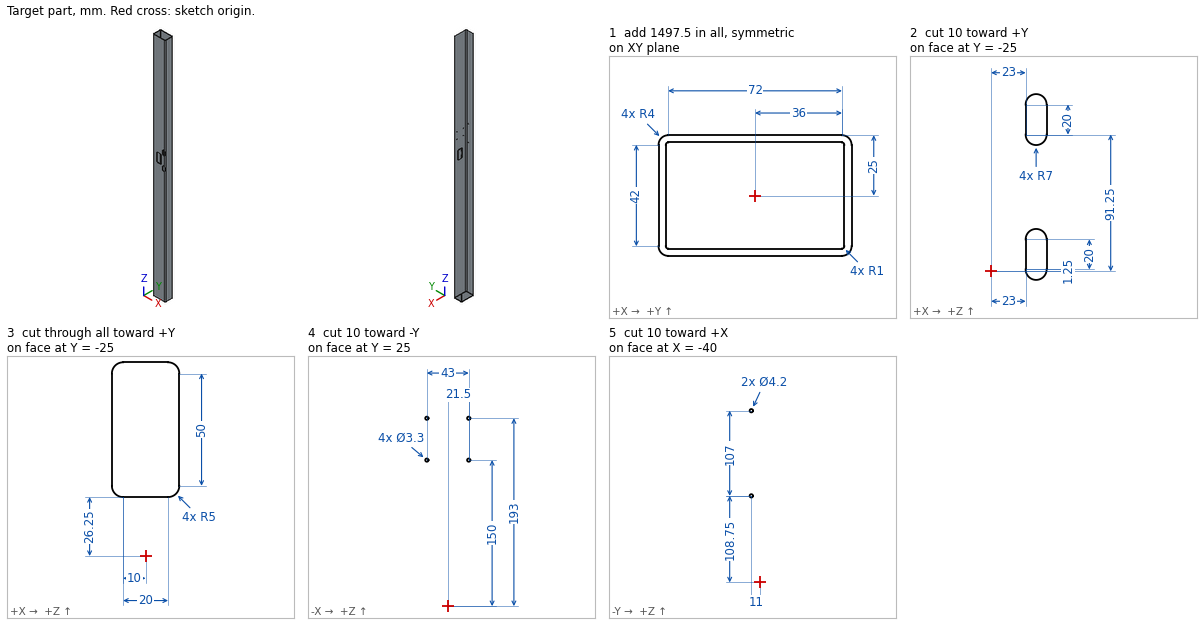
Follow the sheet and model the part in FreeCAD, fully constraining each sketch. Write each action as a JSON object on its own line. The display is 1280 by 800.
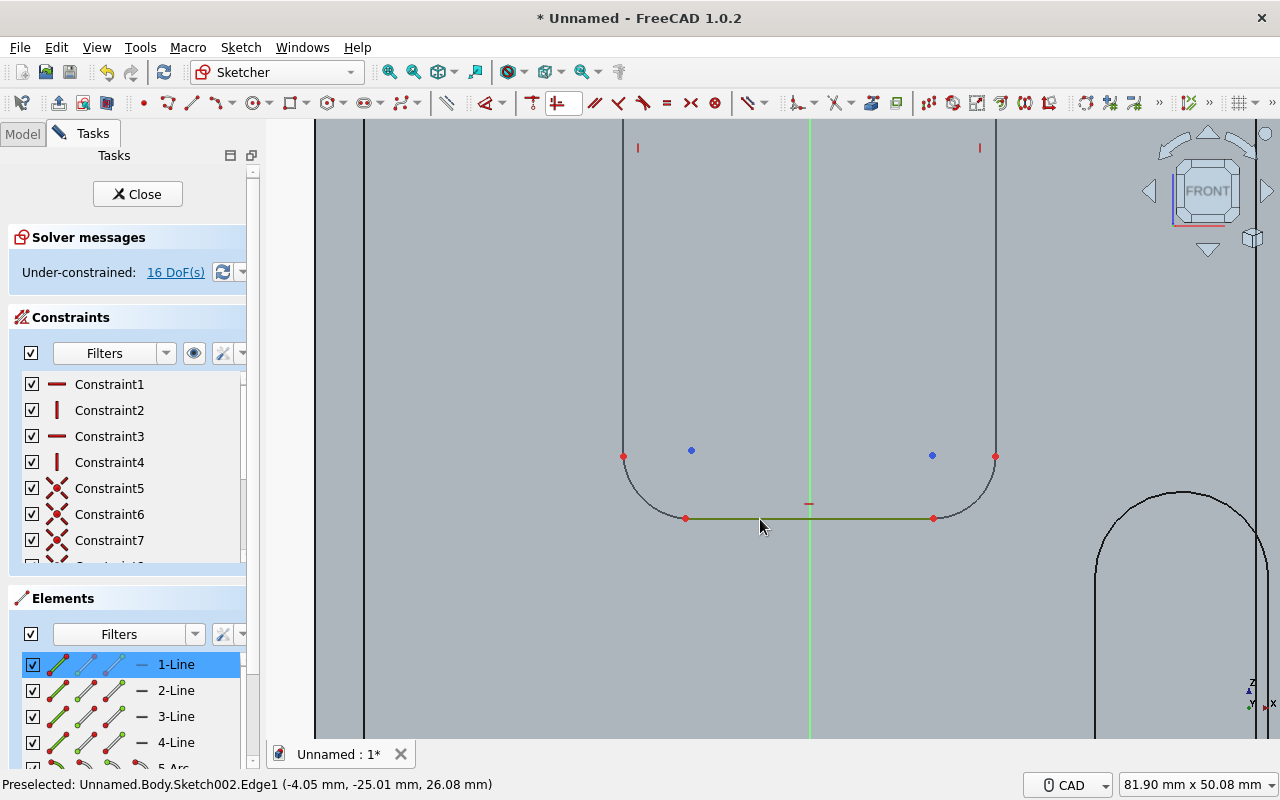
{"action": "left_click", "coordinate": [961, 512]}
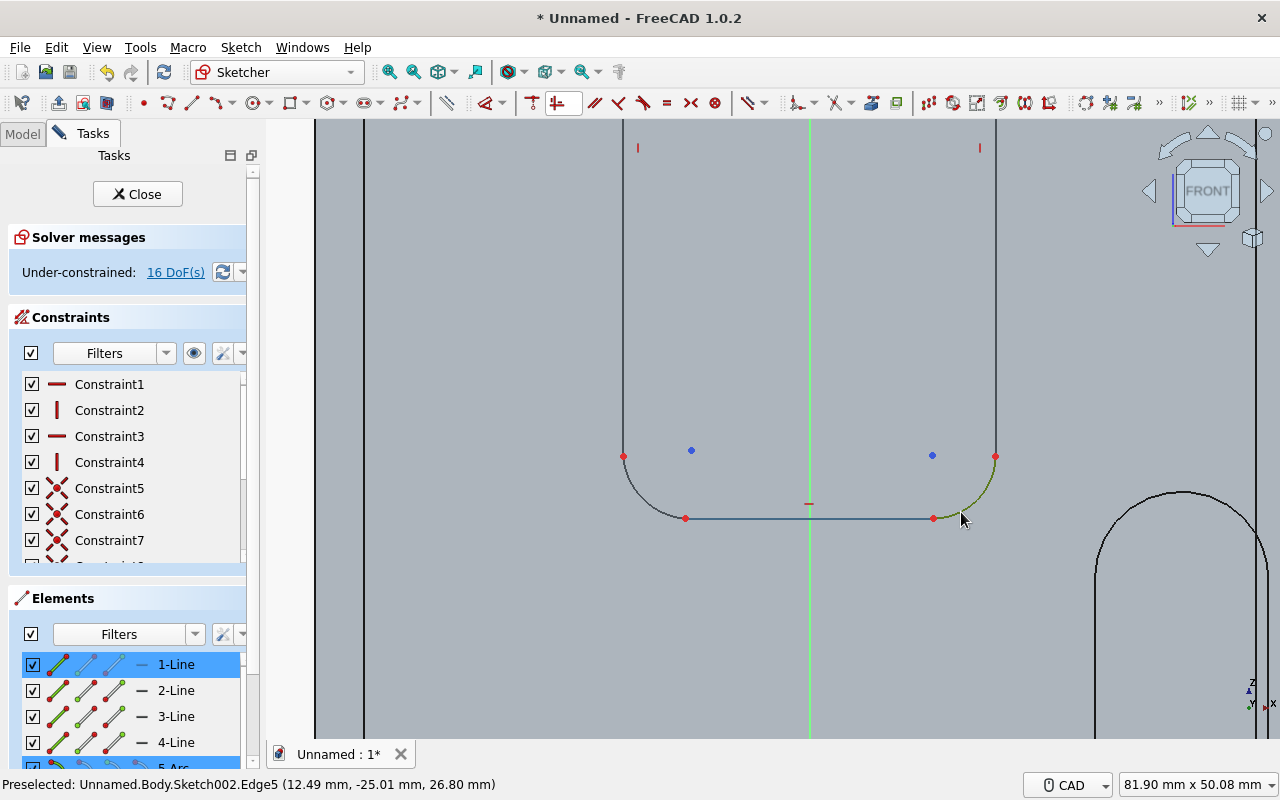
{"action": "key", "text": "t"}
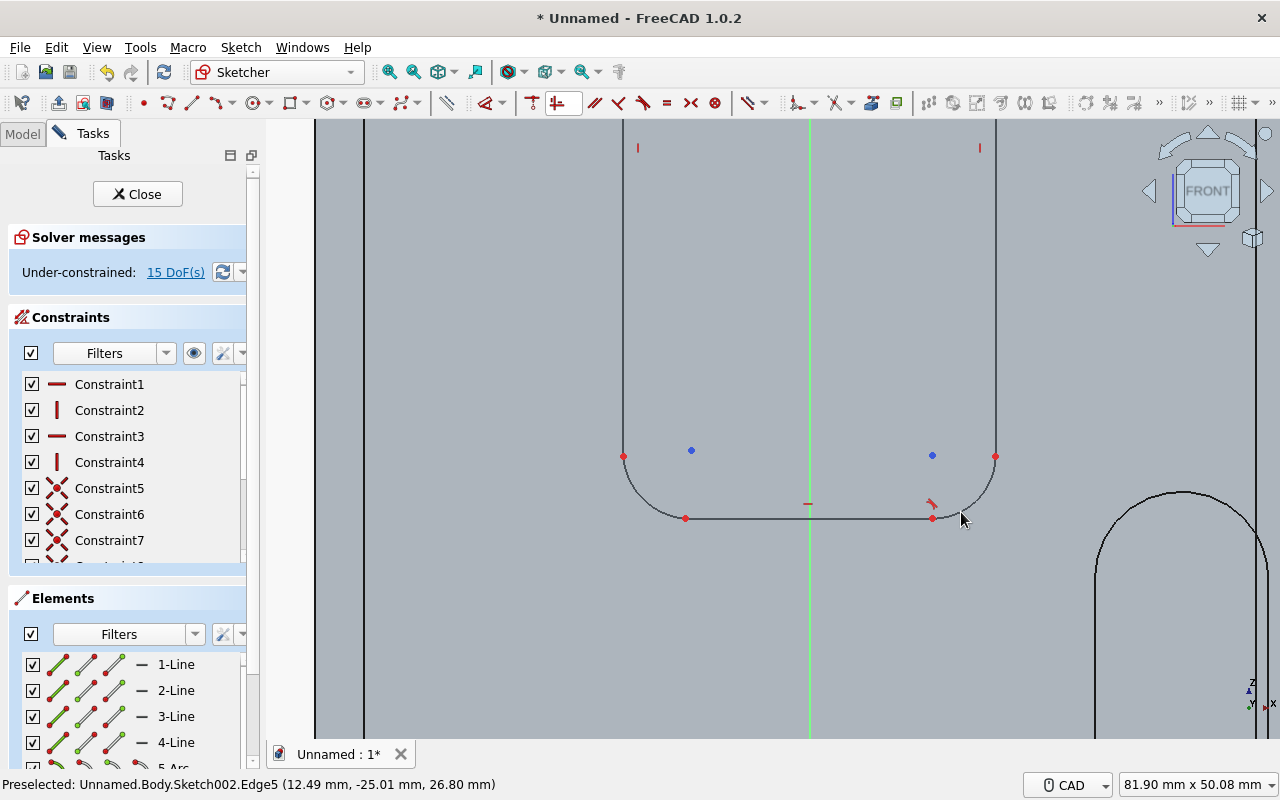
{"action": "left_click", "coordinate": [760, 519]}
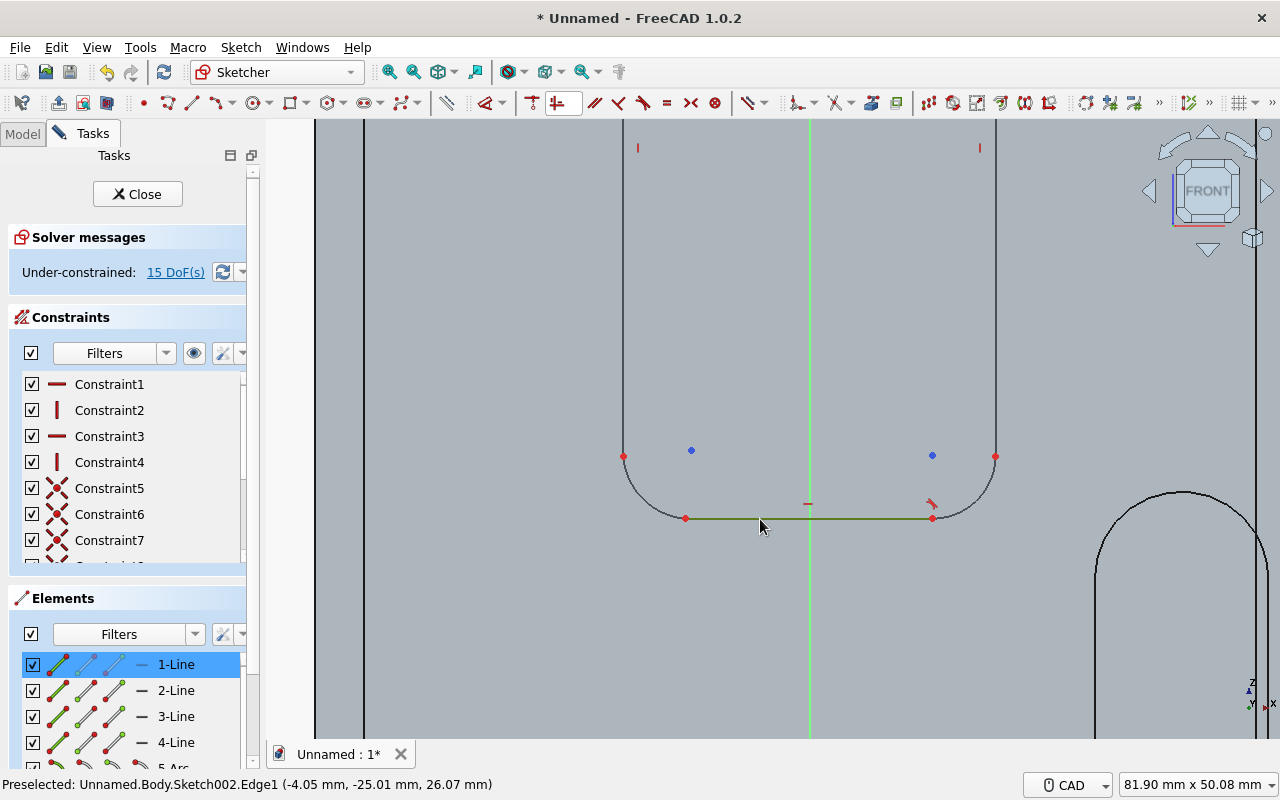
{"action": "left_click", "coordinate": [631, 484]}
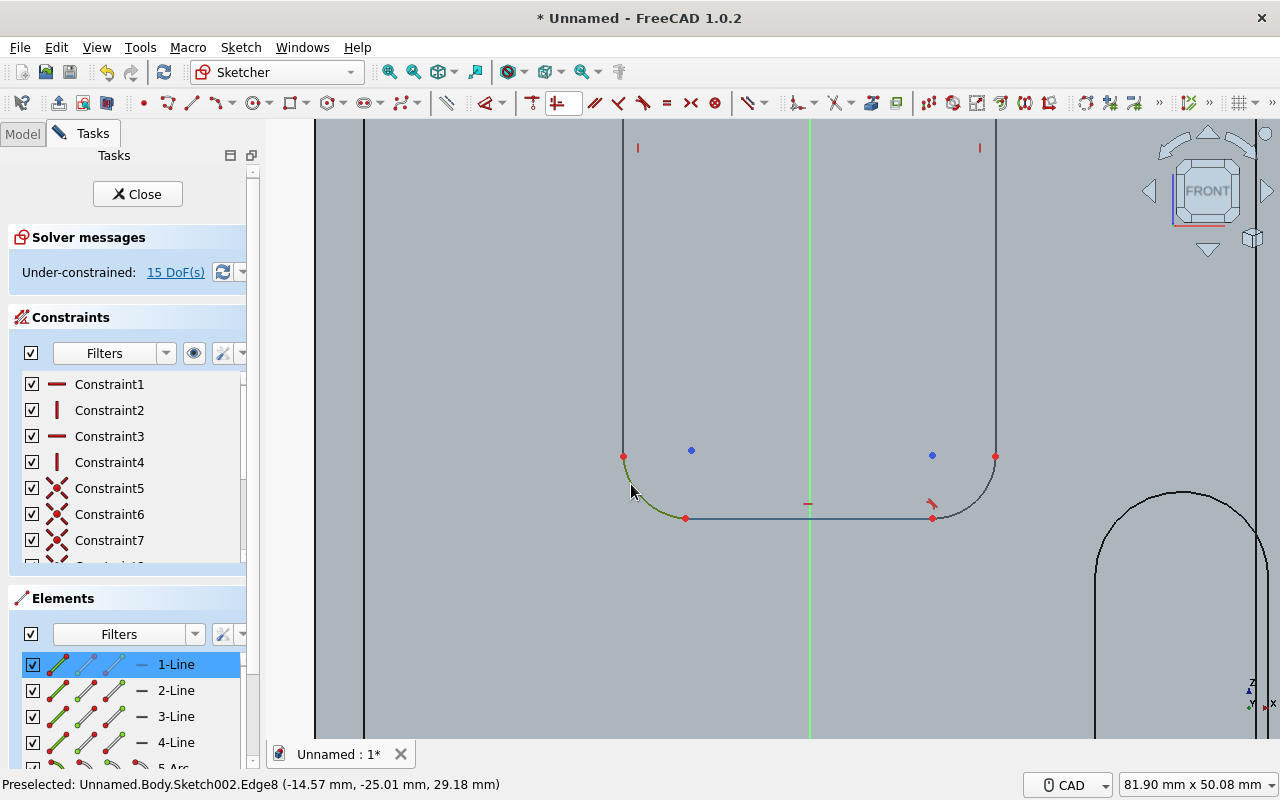
{"action": "left_click", "coordinate": [644, 104]}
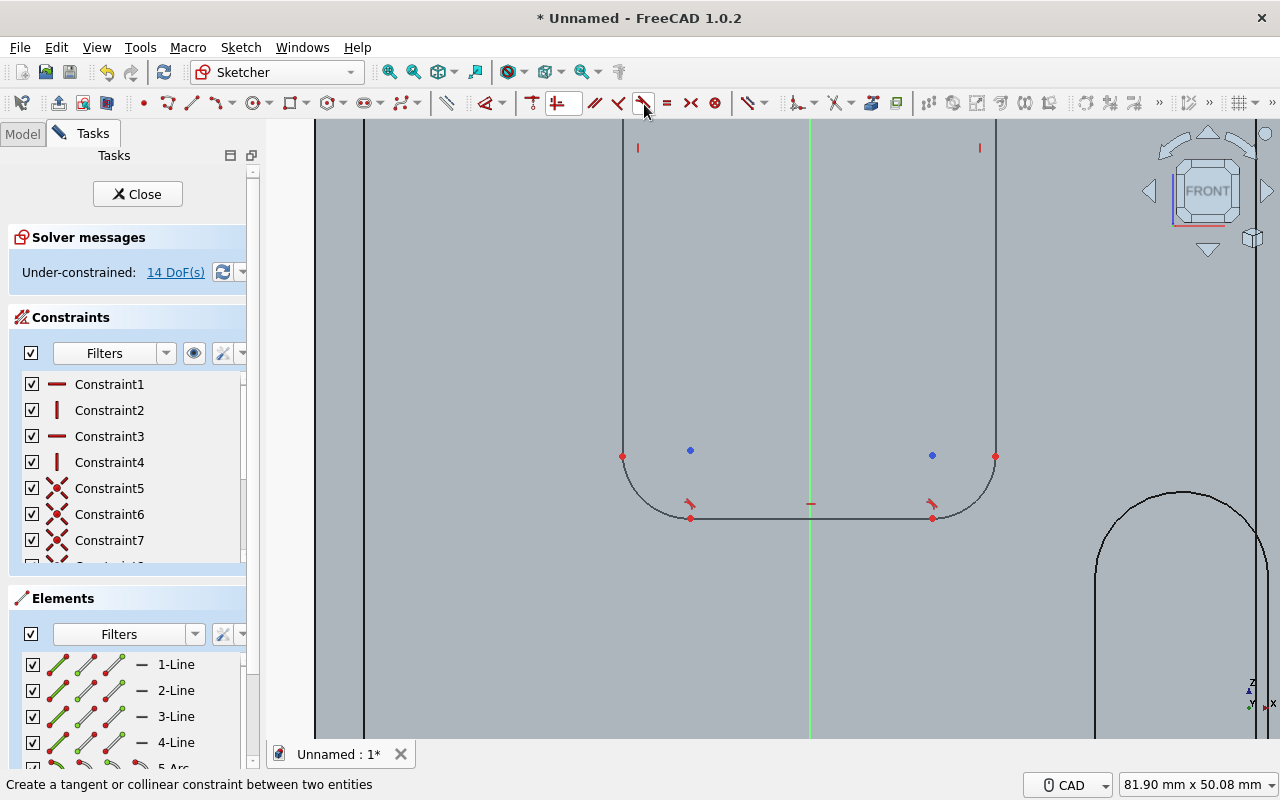
{"action": "left_click", "coordinate": [996, 271]}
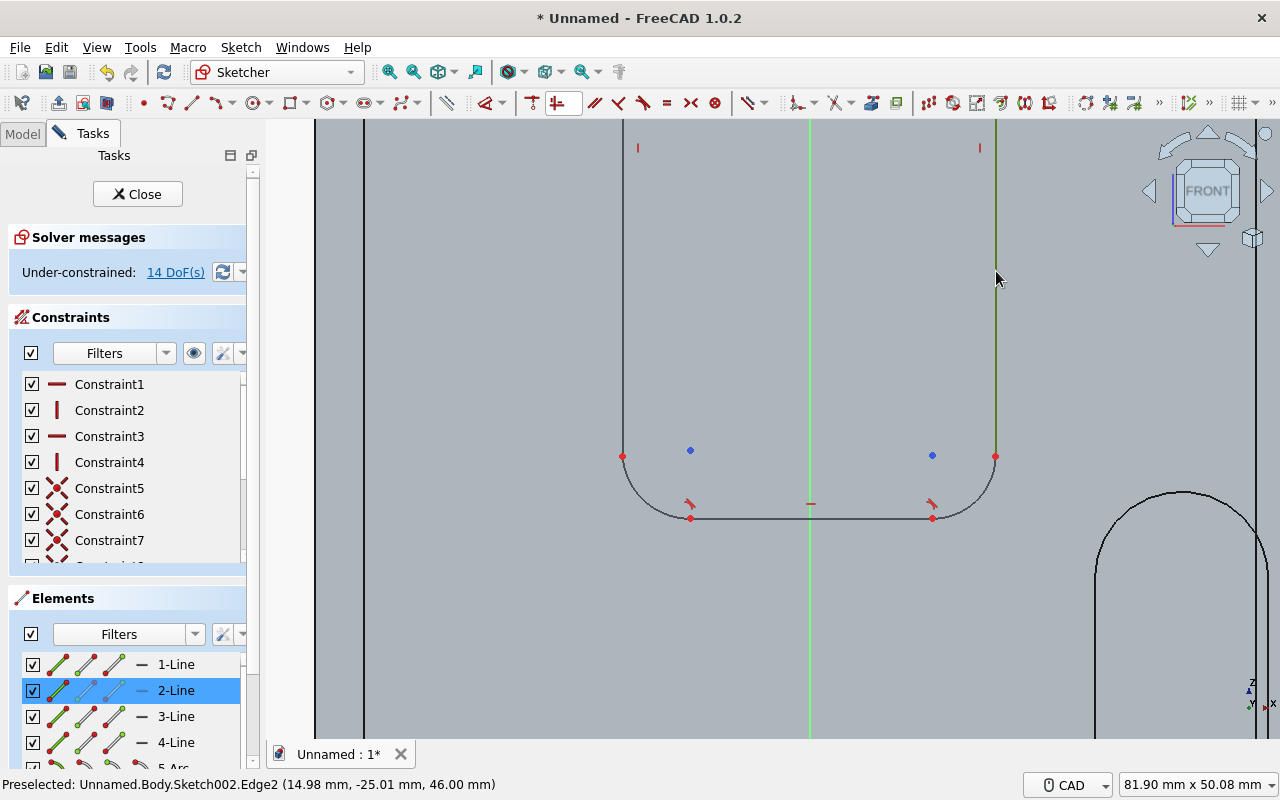
{"action": "left_click", "coordinate": [961, 512]}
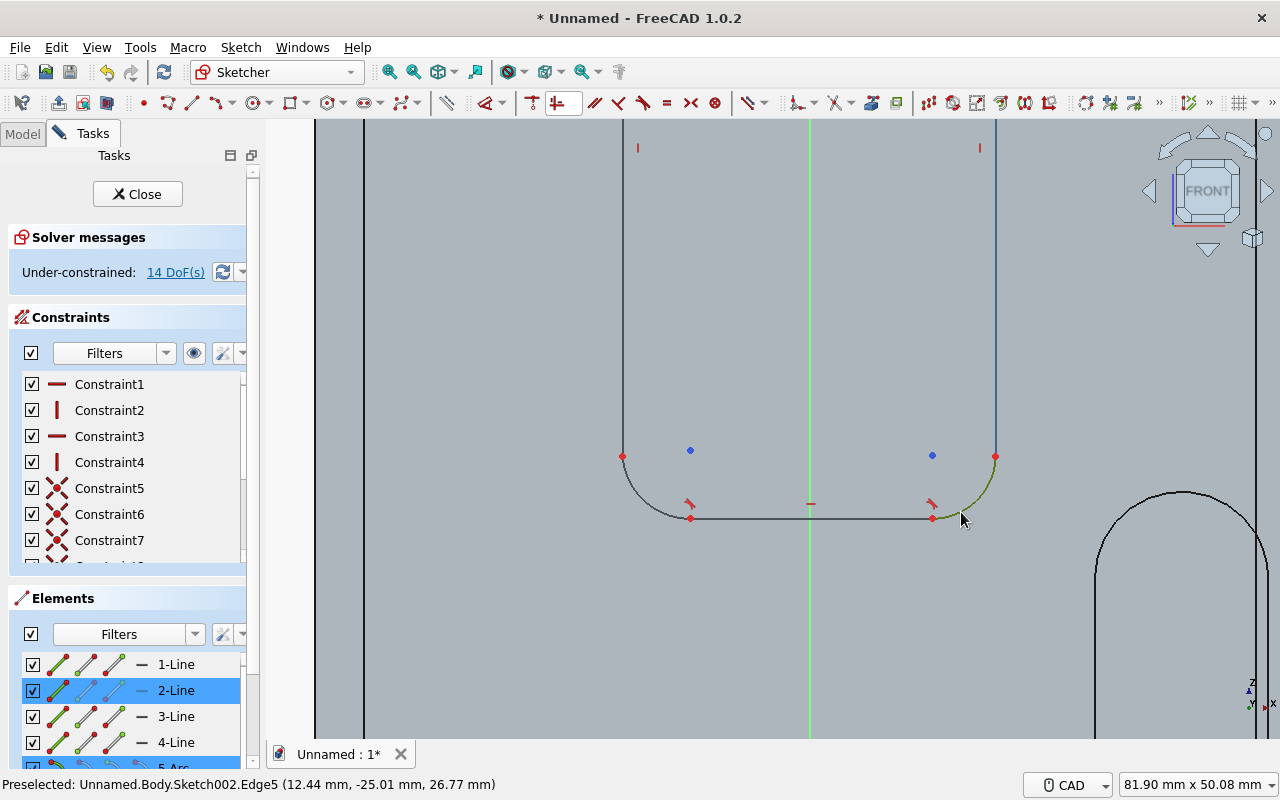
{"action": "key", "text": "t"}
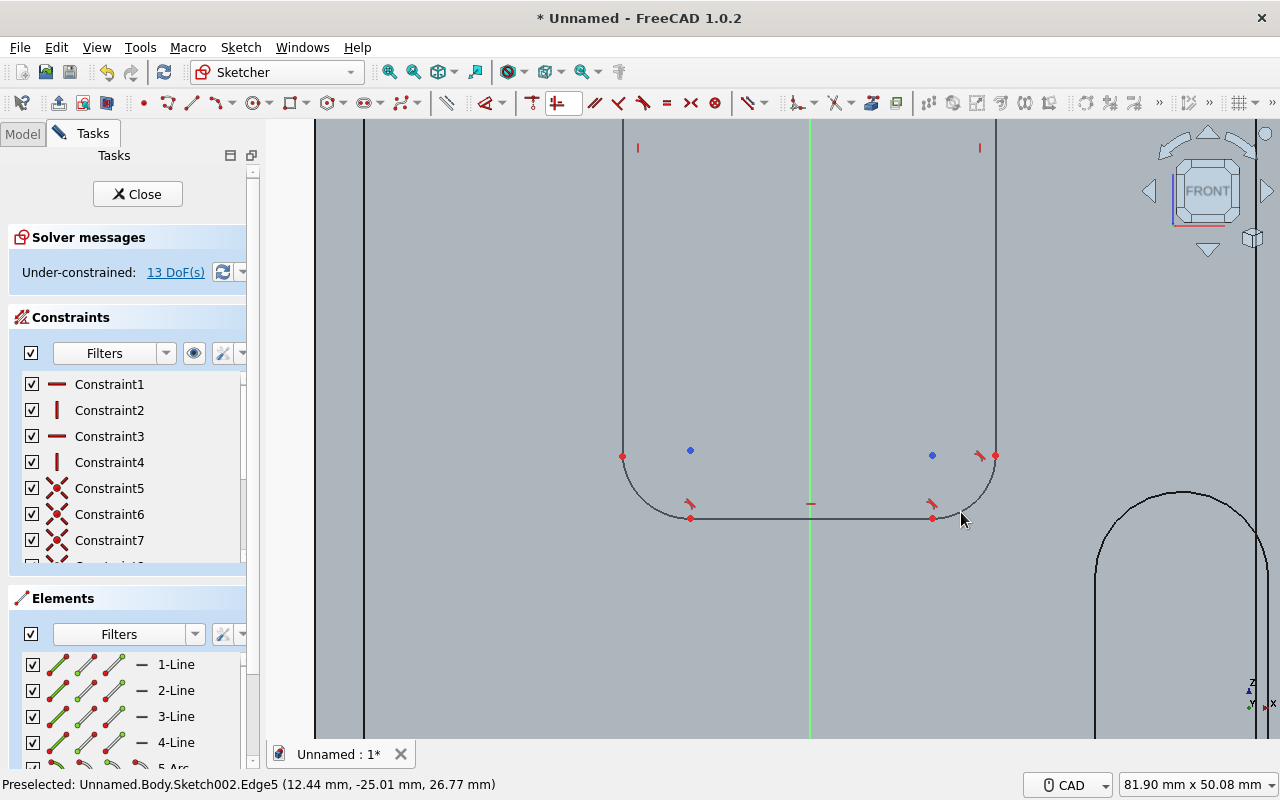
{"action": "left_click", "coordinate": [996, 270]}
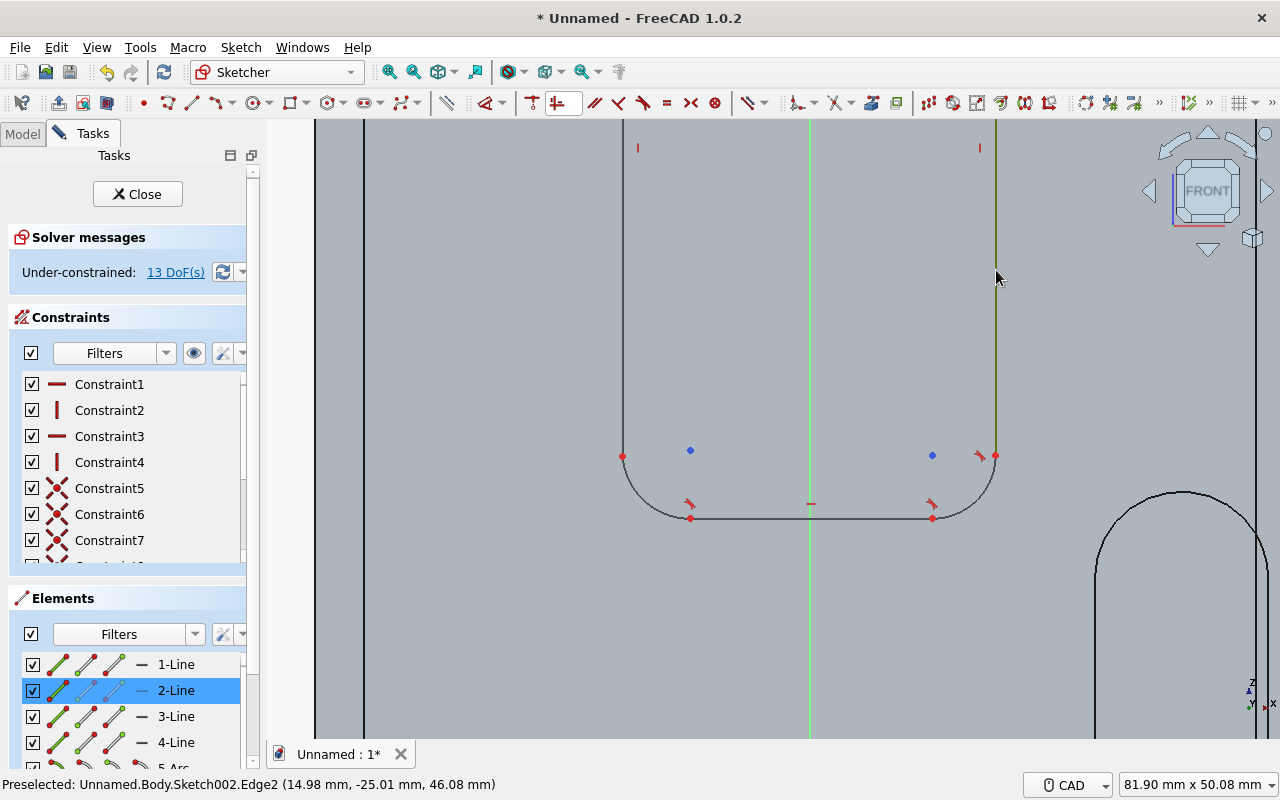
{"action": "scroll", "coordinate": [643, 500], "scroll_direction": "down", "scroll_amount": 5}